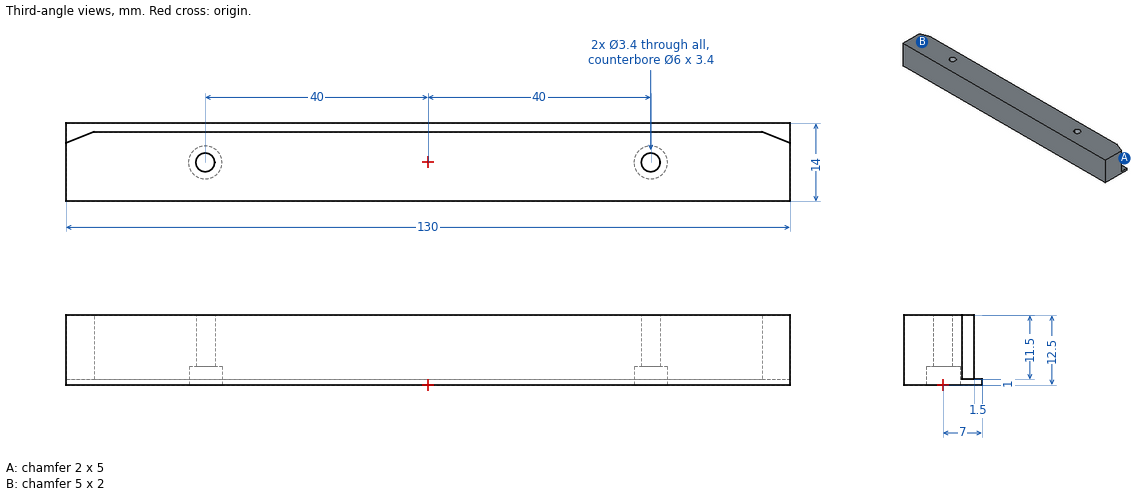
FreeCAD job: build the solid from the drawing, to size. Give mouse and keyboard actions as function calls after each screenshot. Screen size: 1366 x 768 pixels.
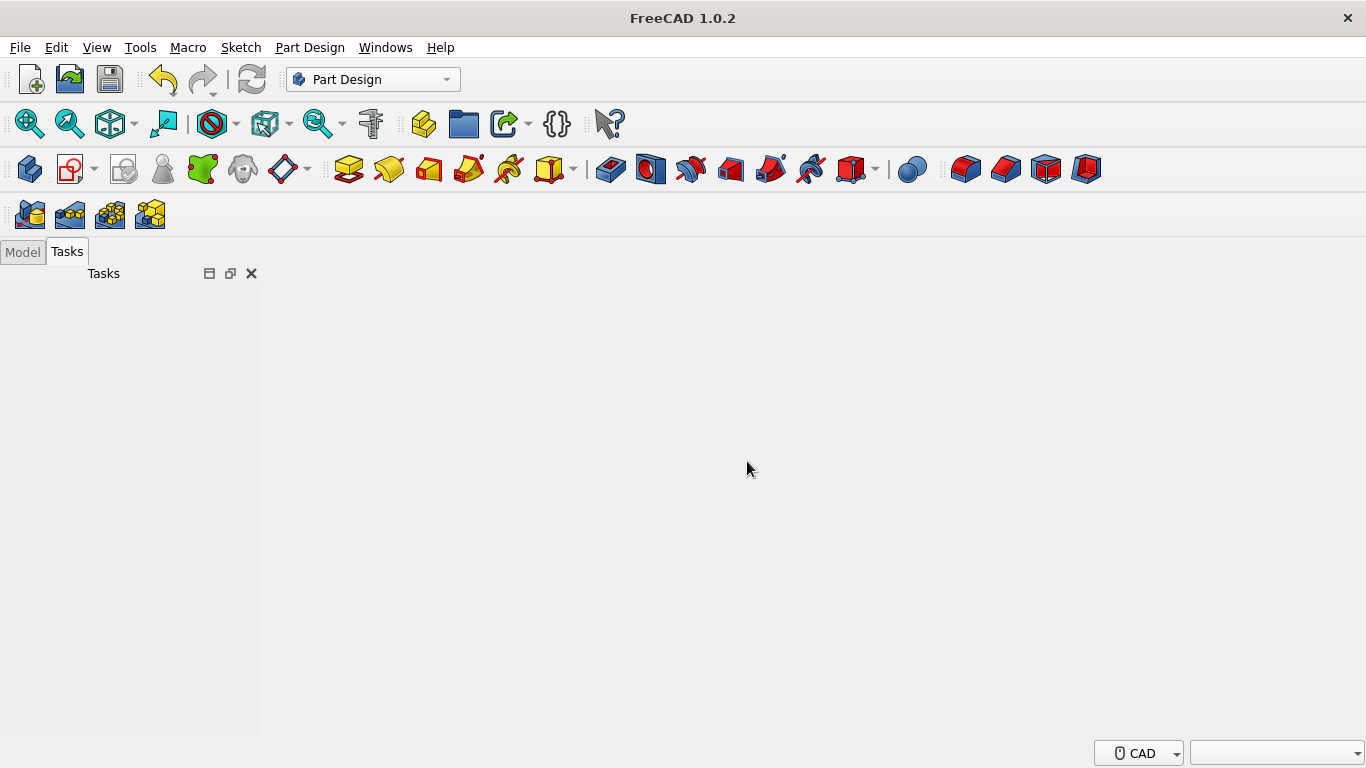
click(30, 80)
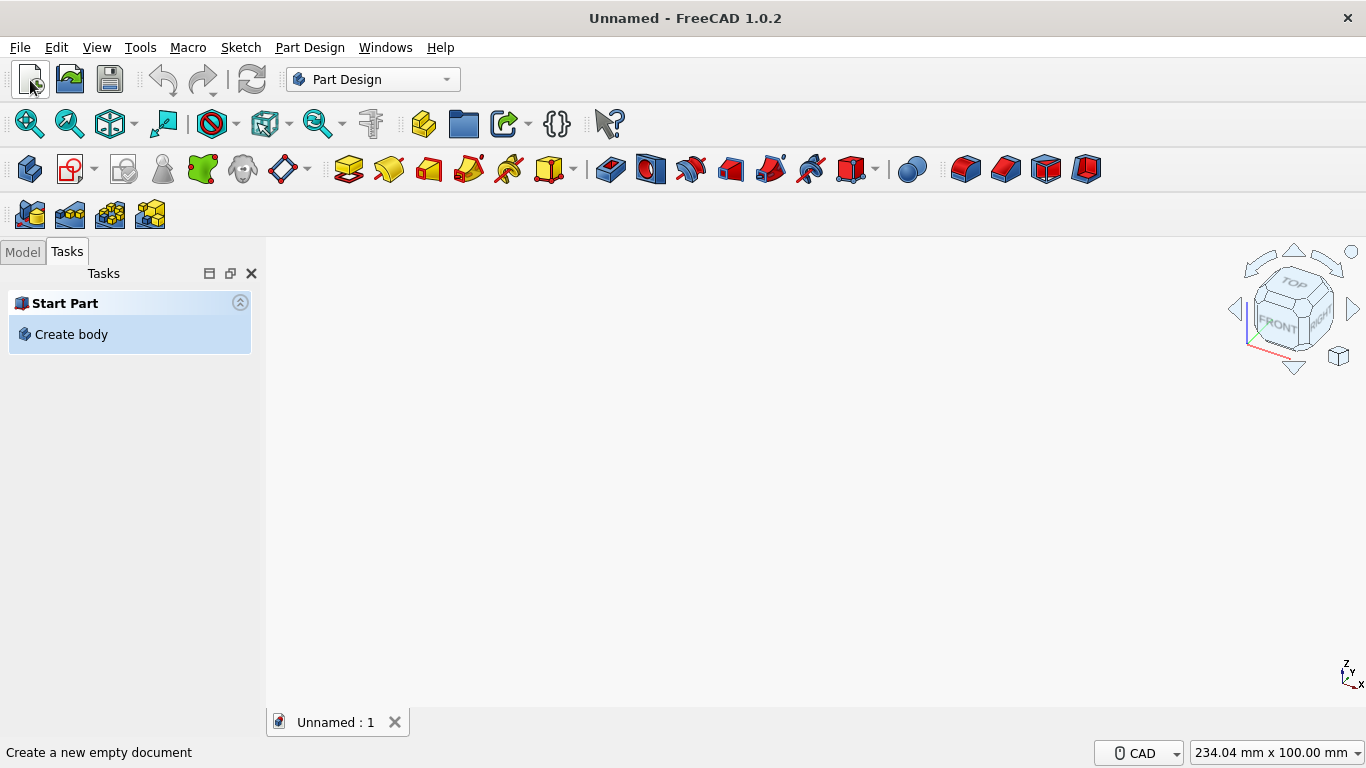
click(70, 170)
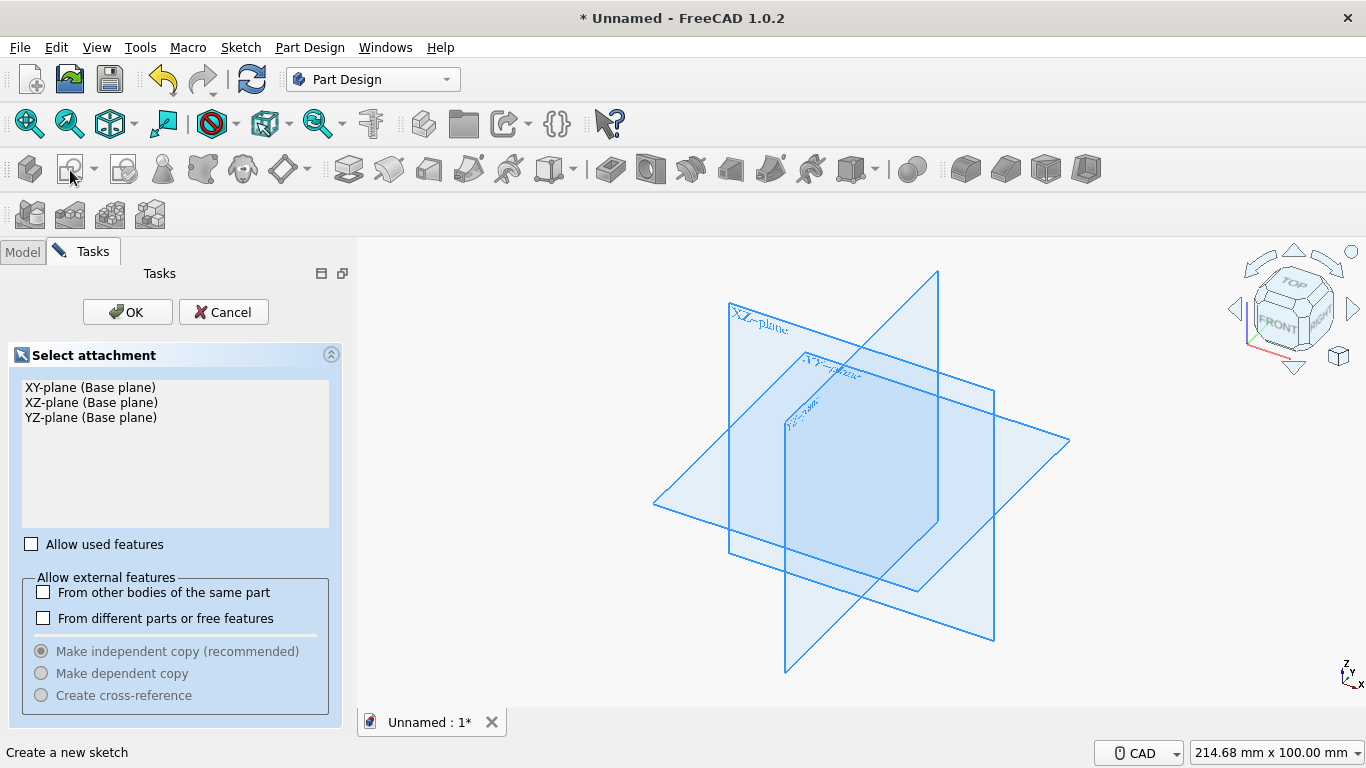
click(82, 388)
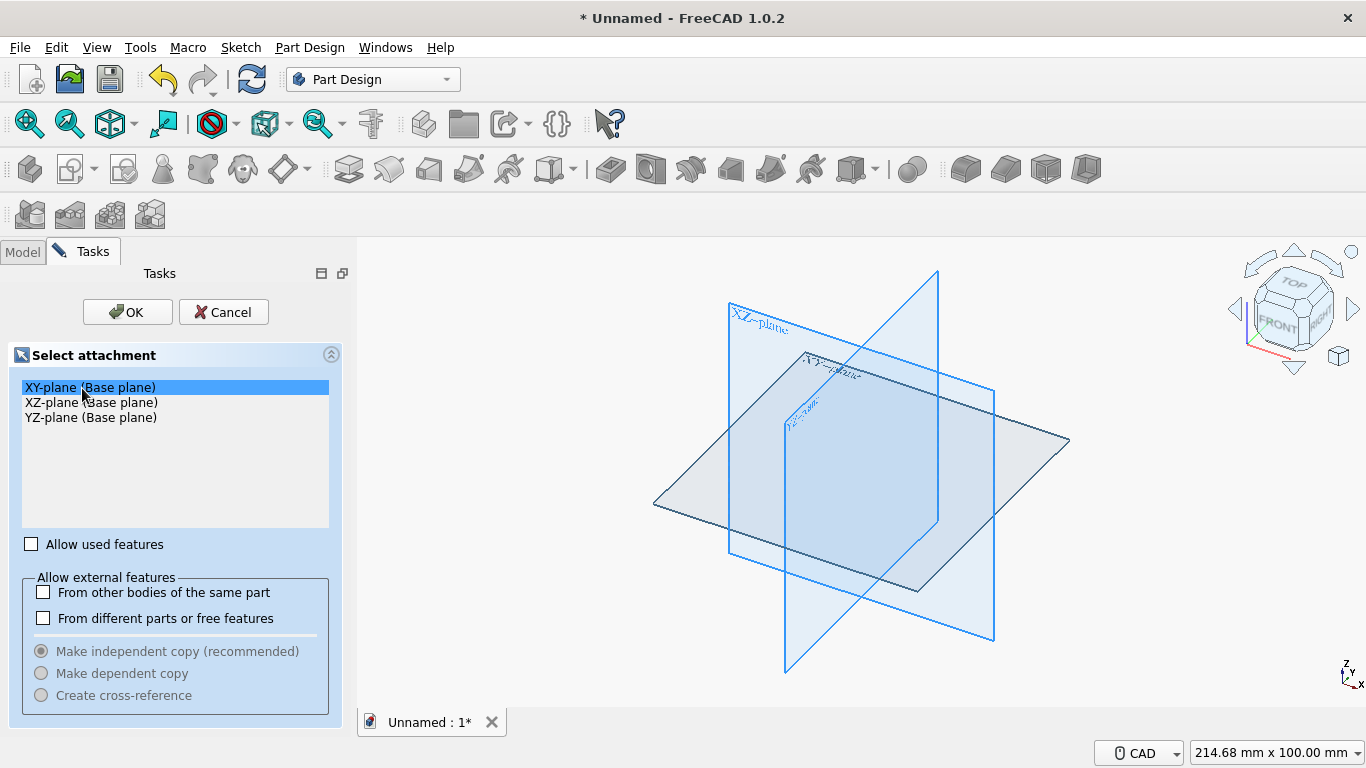
click(128, 312)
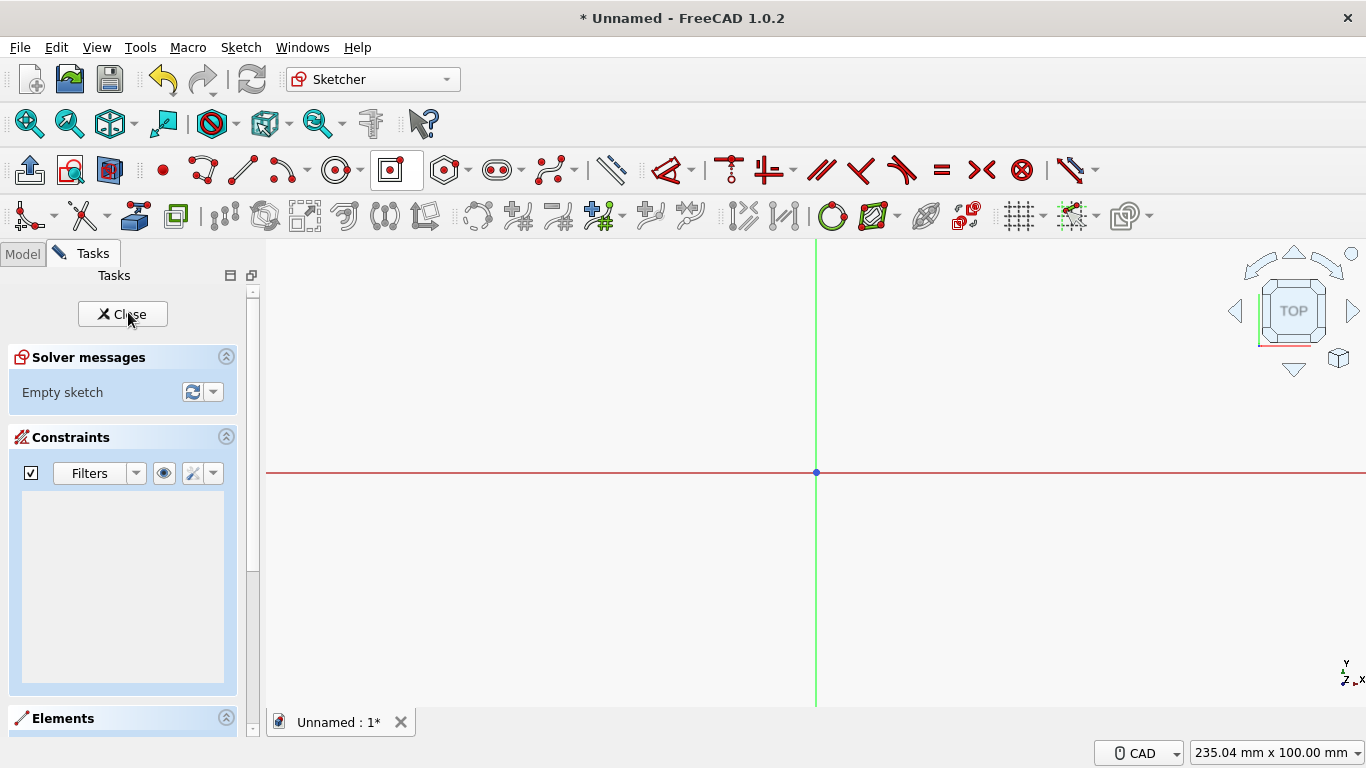
click(390, 170)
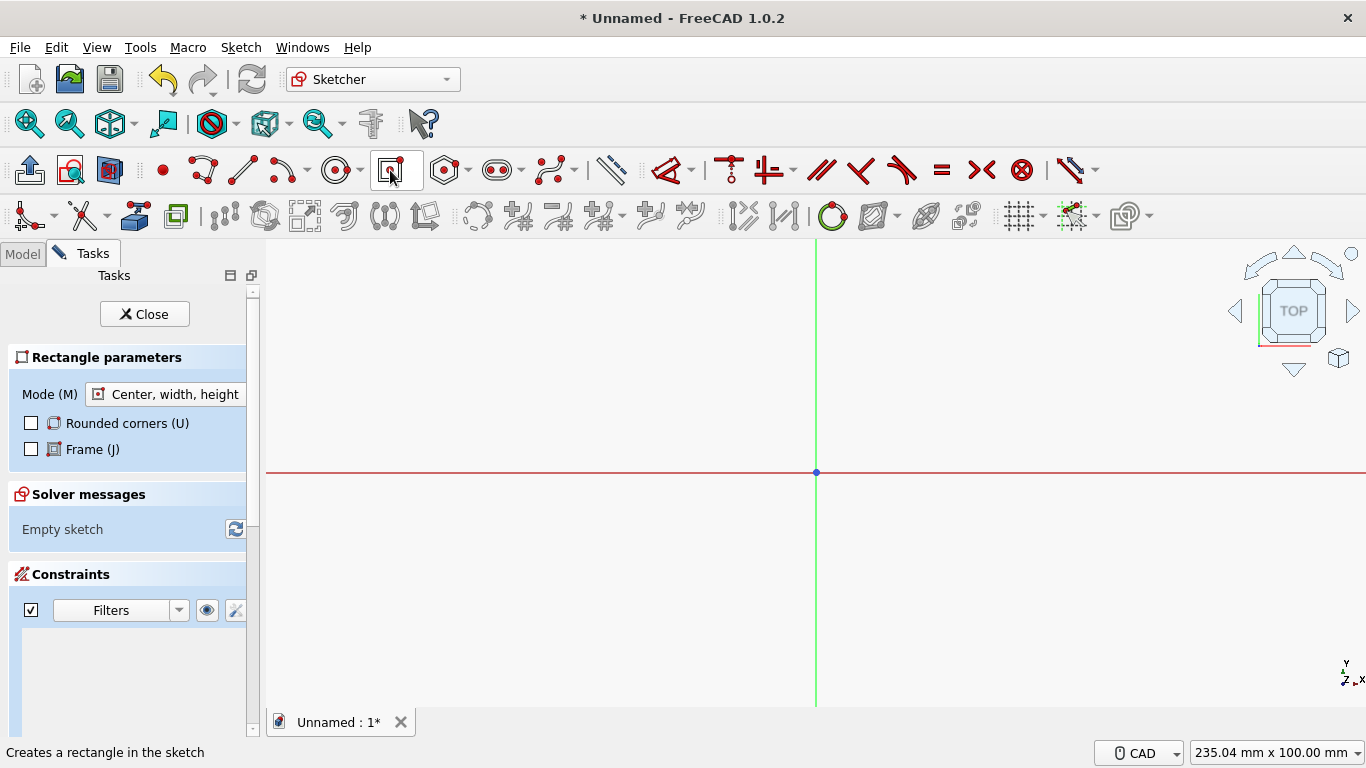
click(816, 473)
click(1120, 440)
key(Escape)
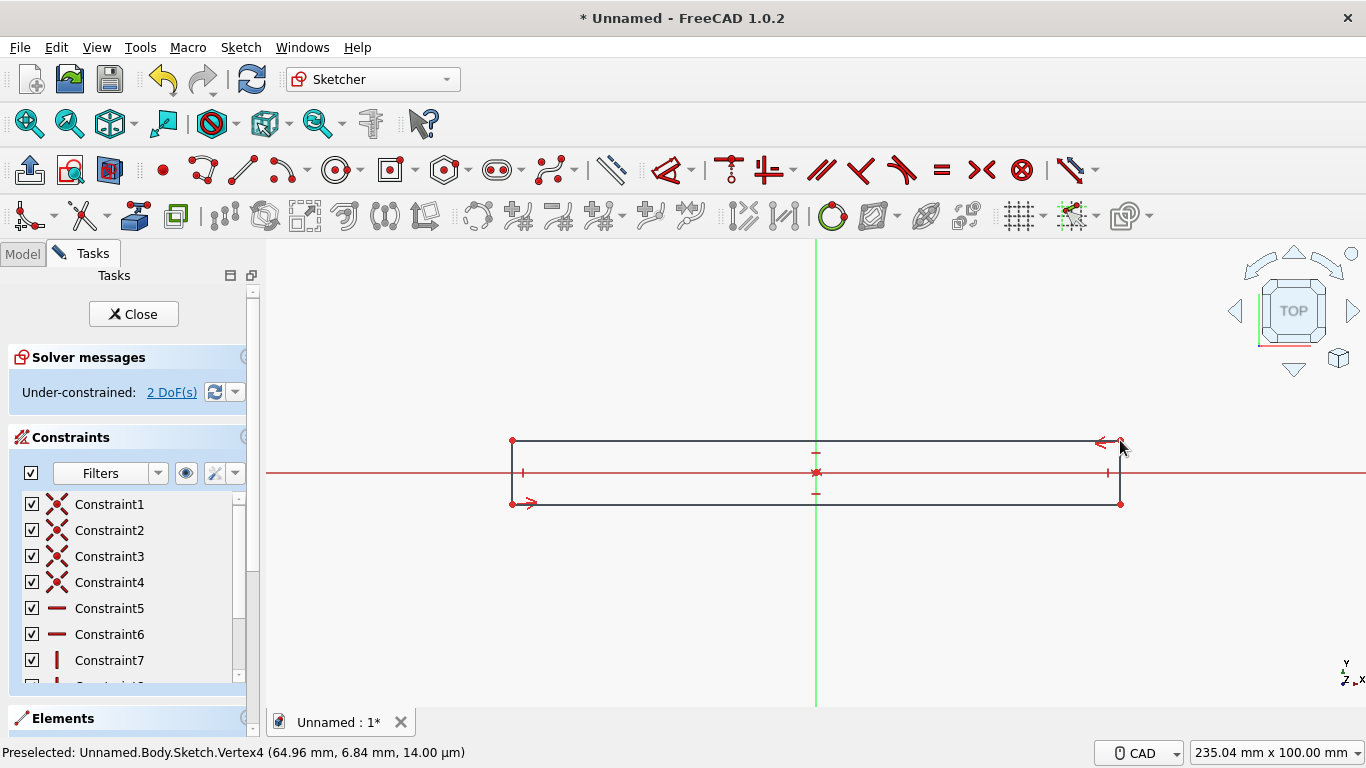
click(1120, 486)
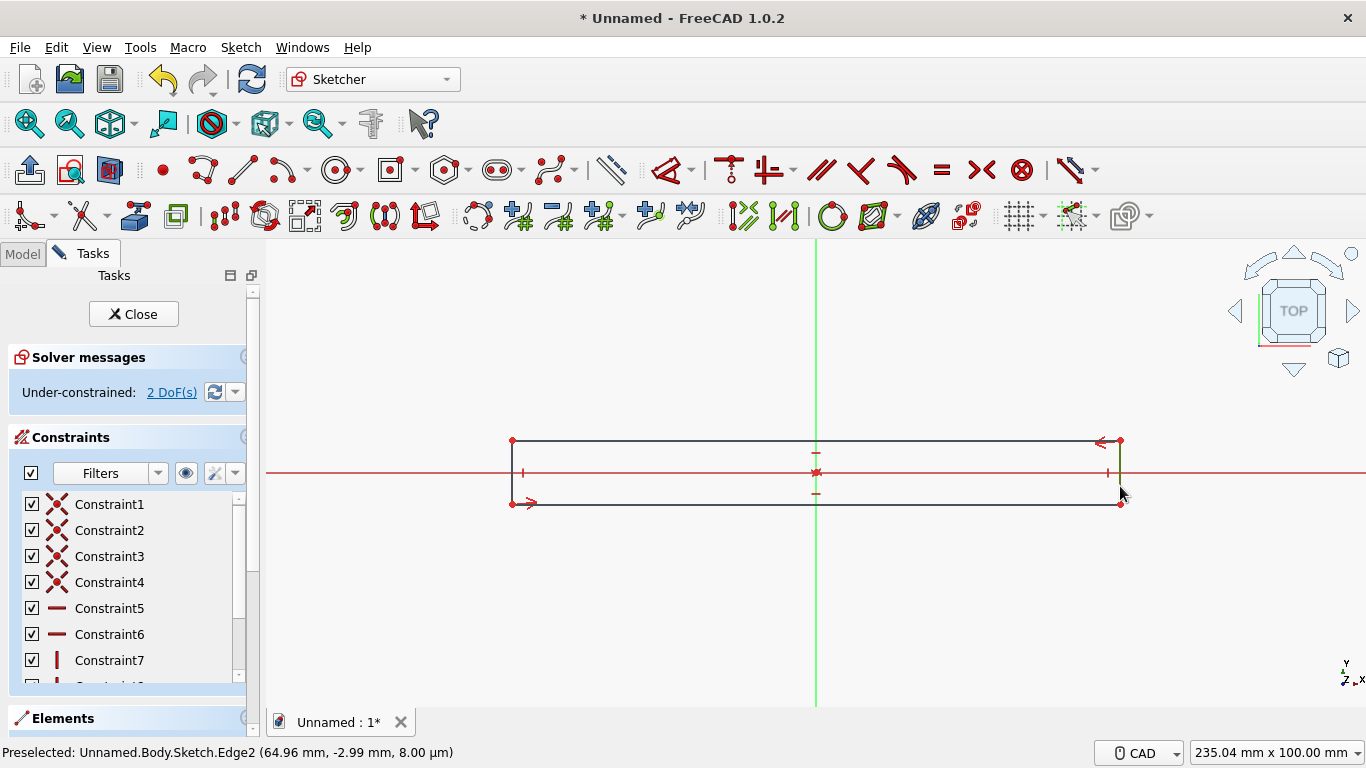
key(i)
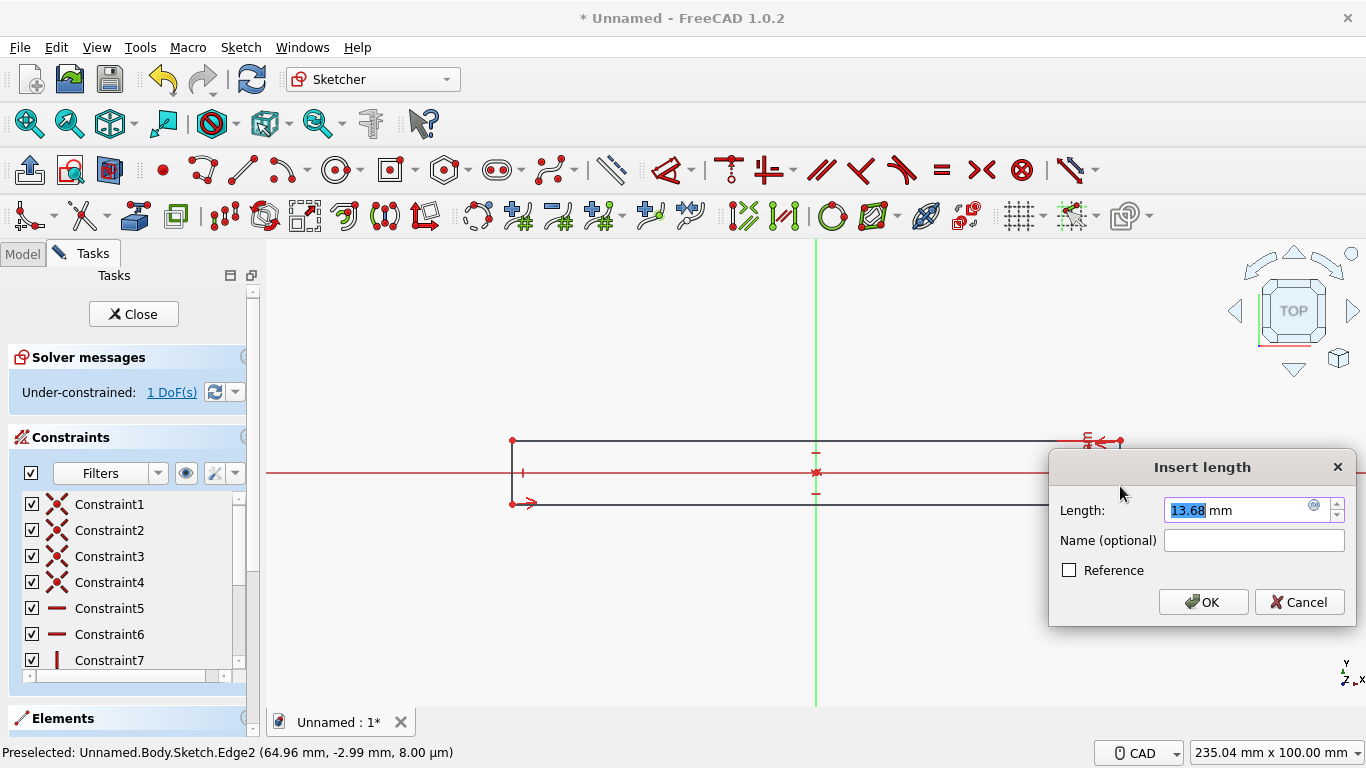
text(14)
key(Return)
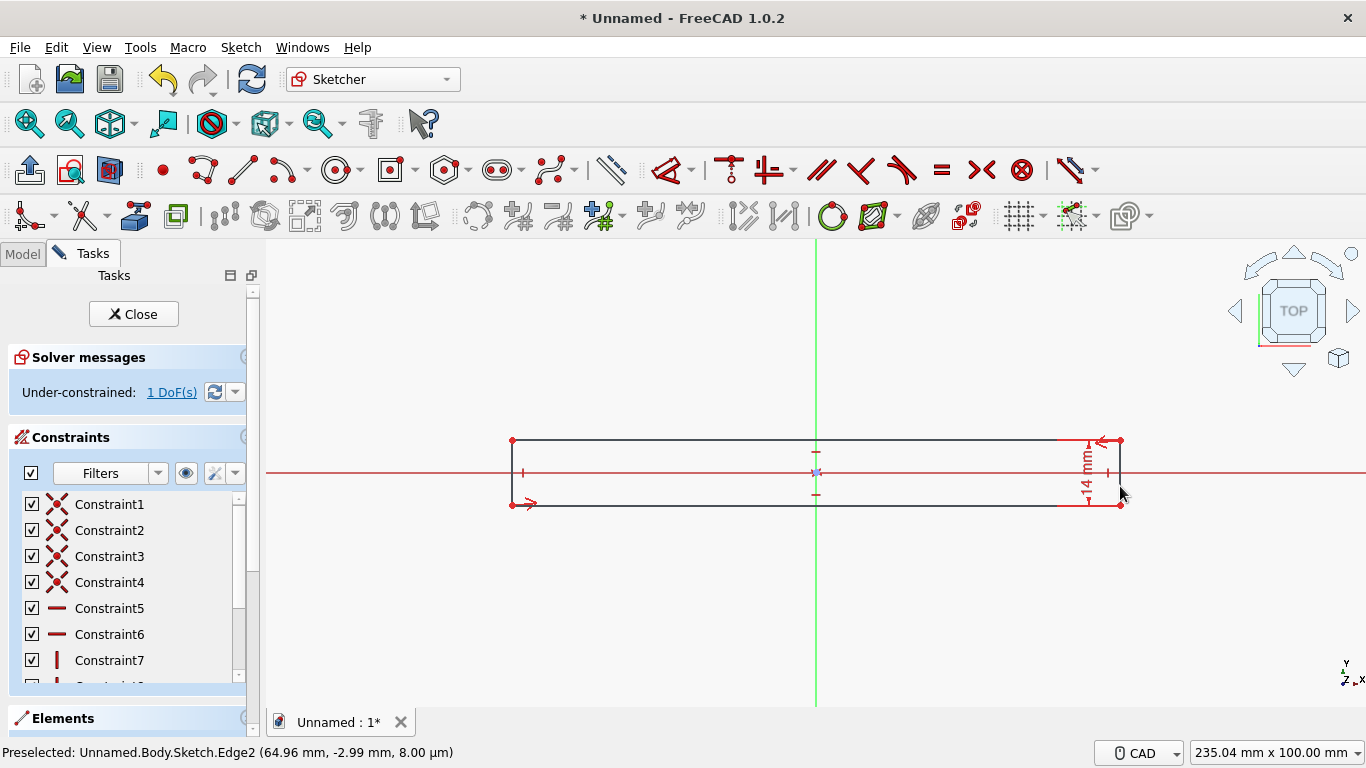
click(694, 506)